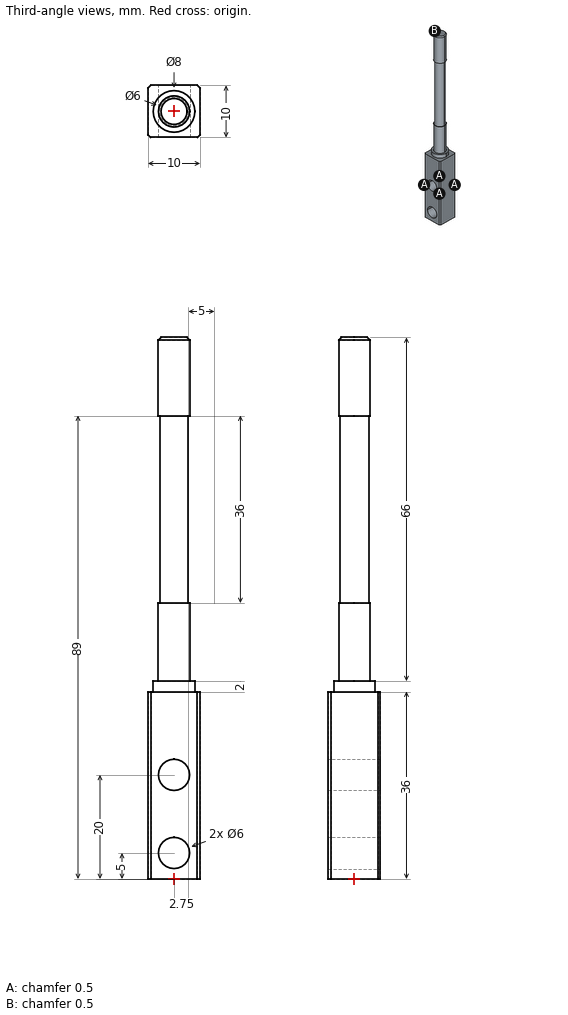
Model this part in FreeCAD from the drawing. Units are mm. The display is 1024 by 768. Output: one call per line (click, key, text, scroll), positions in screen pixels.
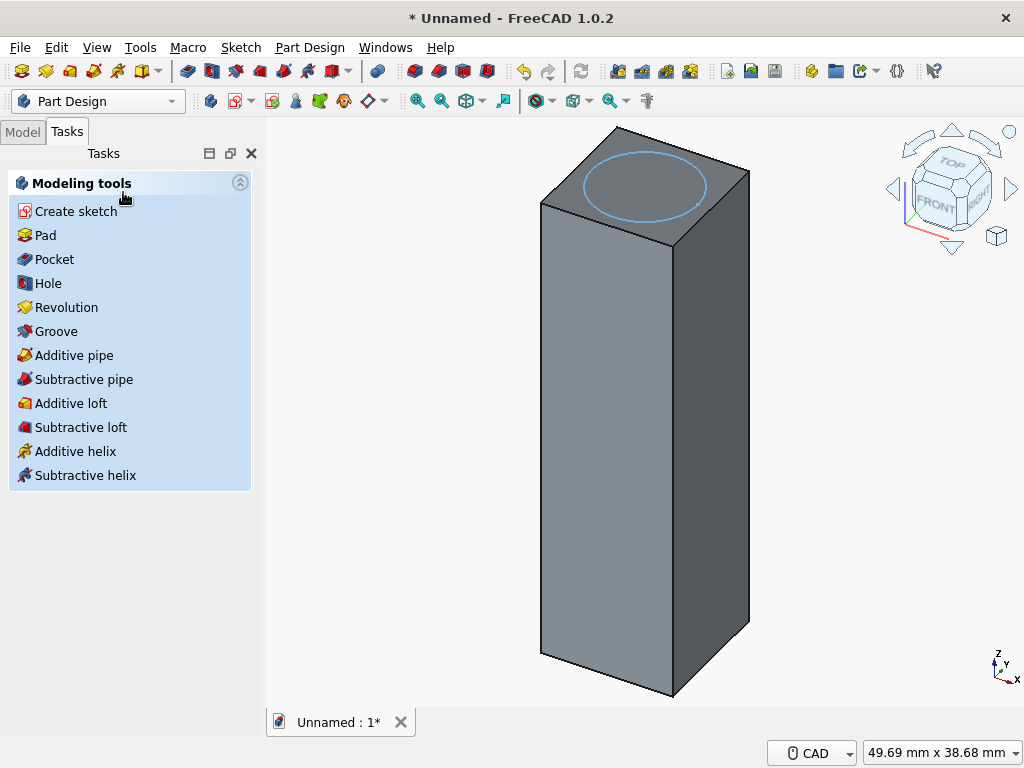
click(22, 72)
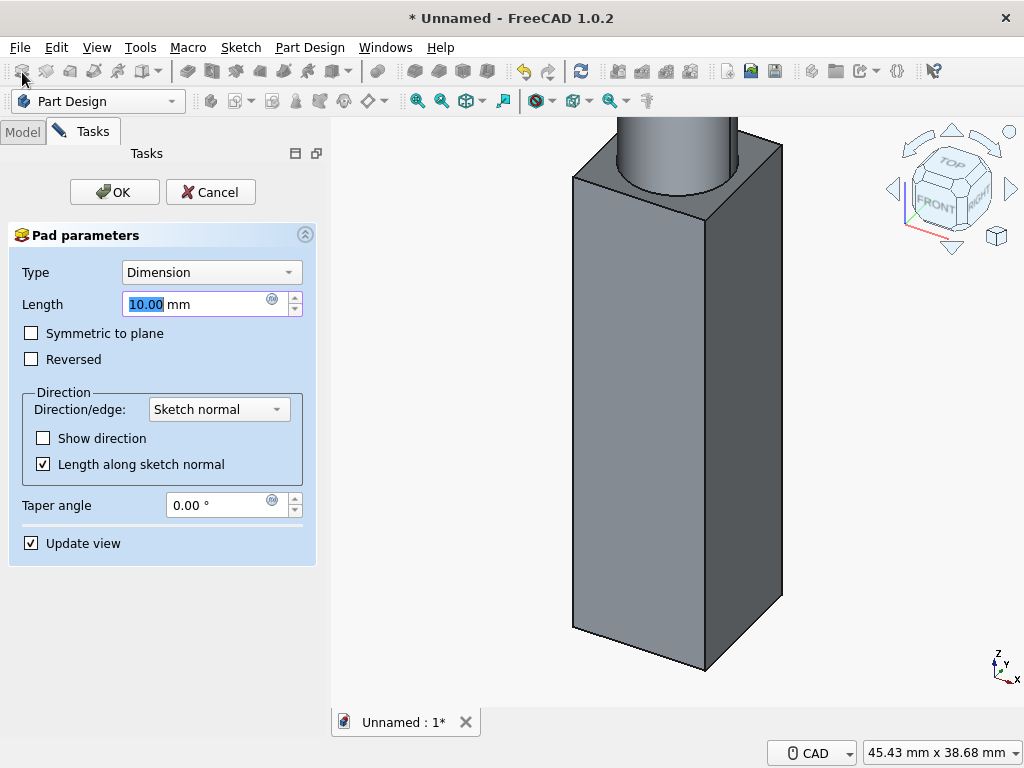
text(2)
key(Tab)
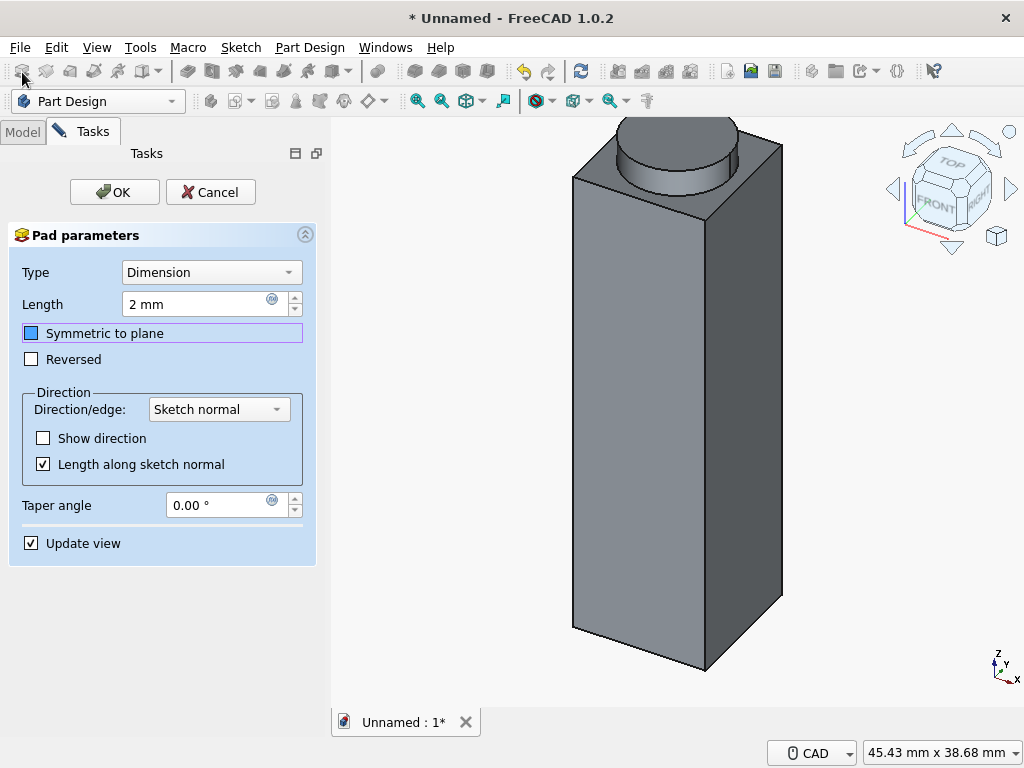
click(115, 192)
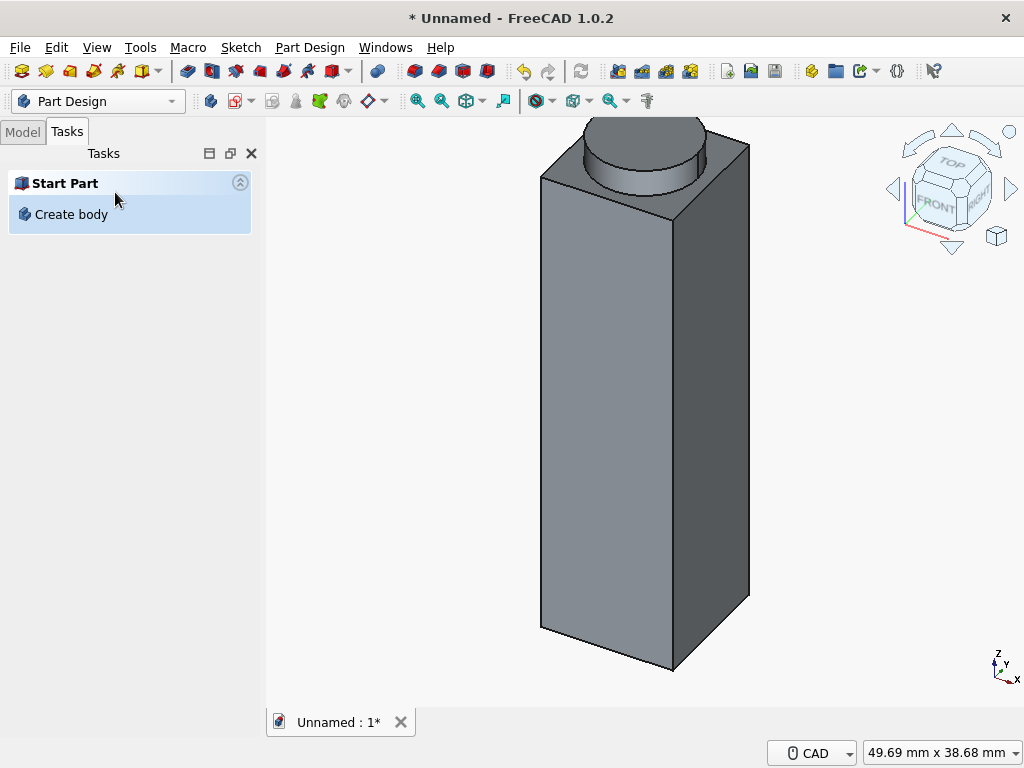
click(418, 102)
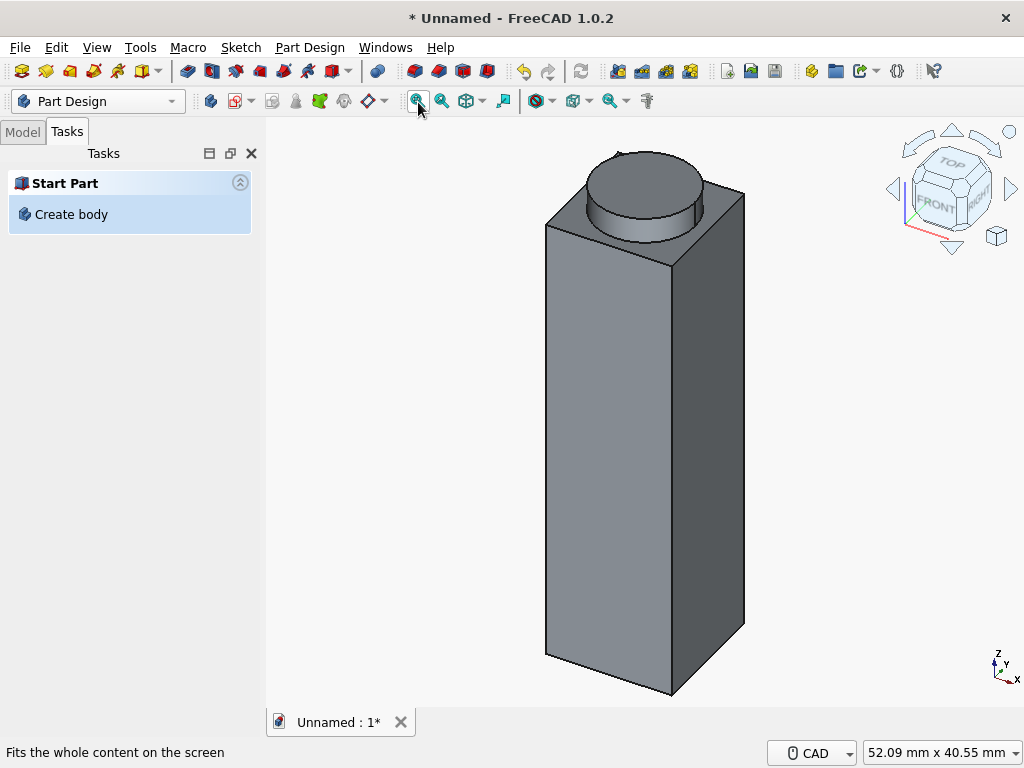
click(645, 185)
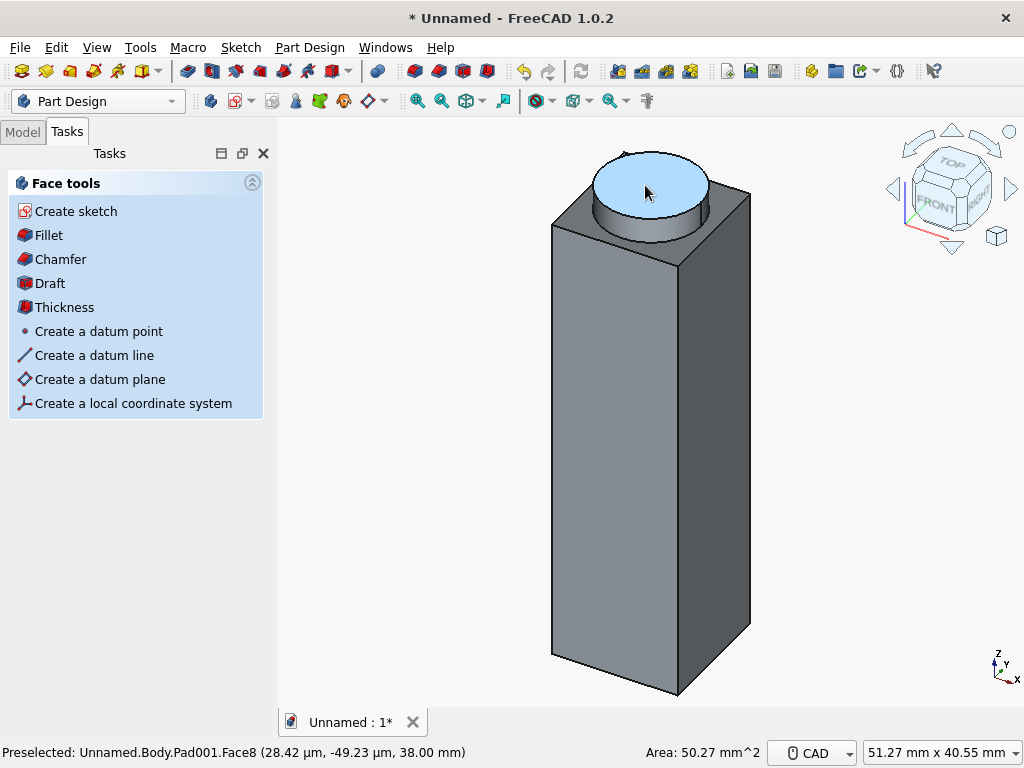
click(236, 102)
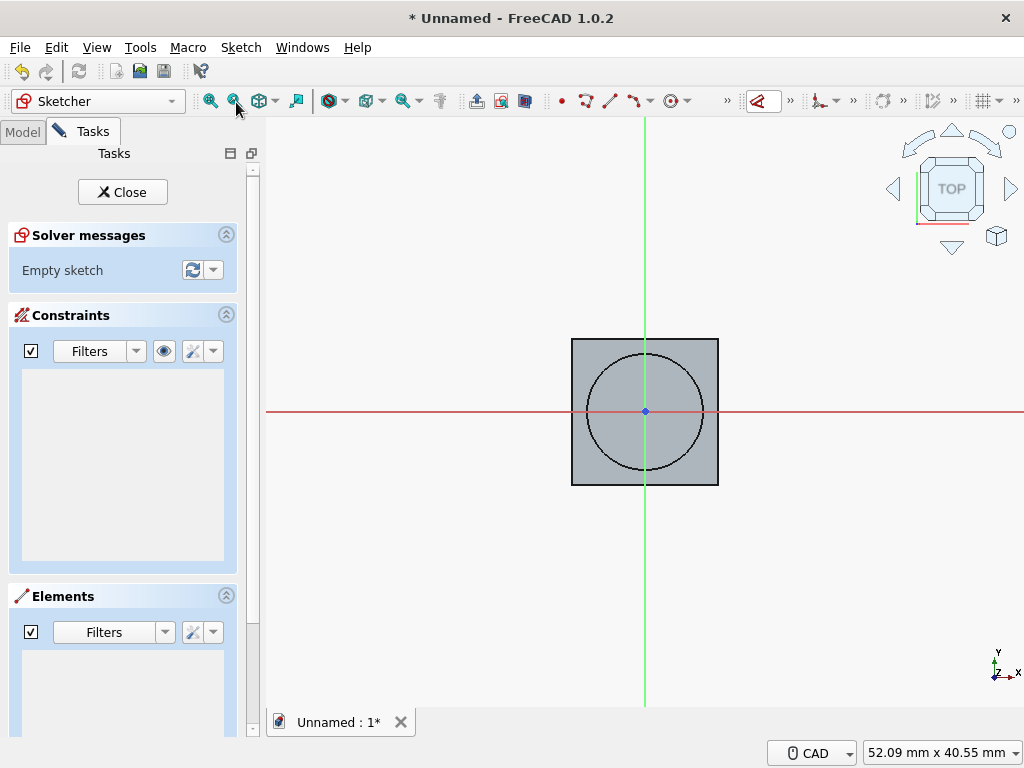
scroll(667, 412, up, 7)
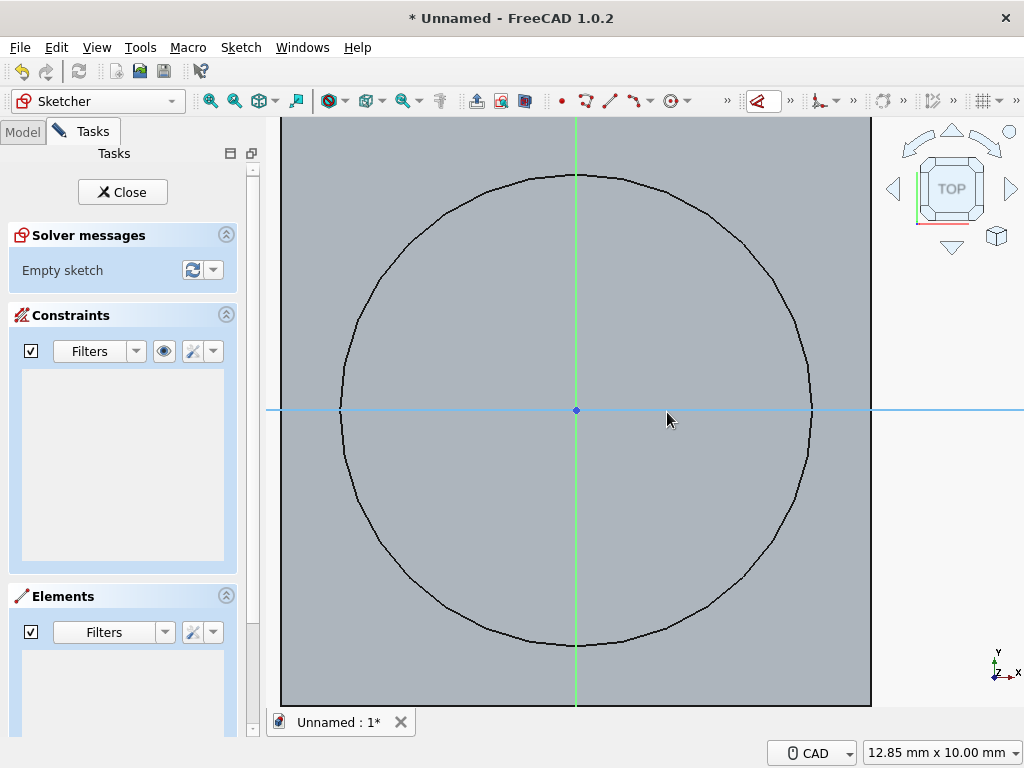
key(g)
key(c)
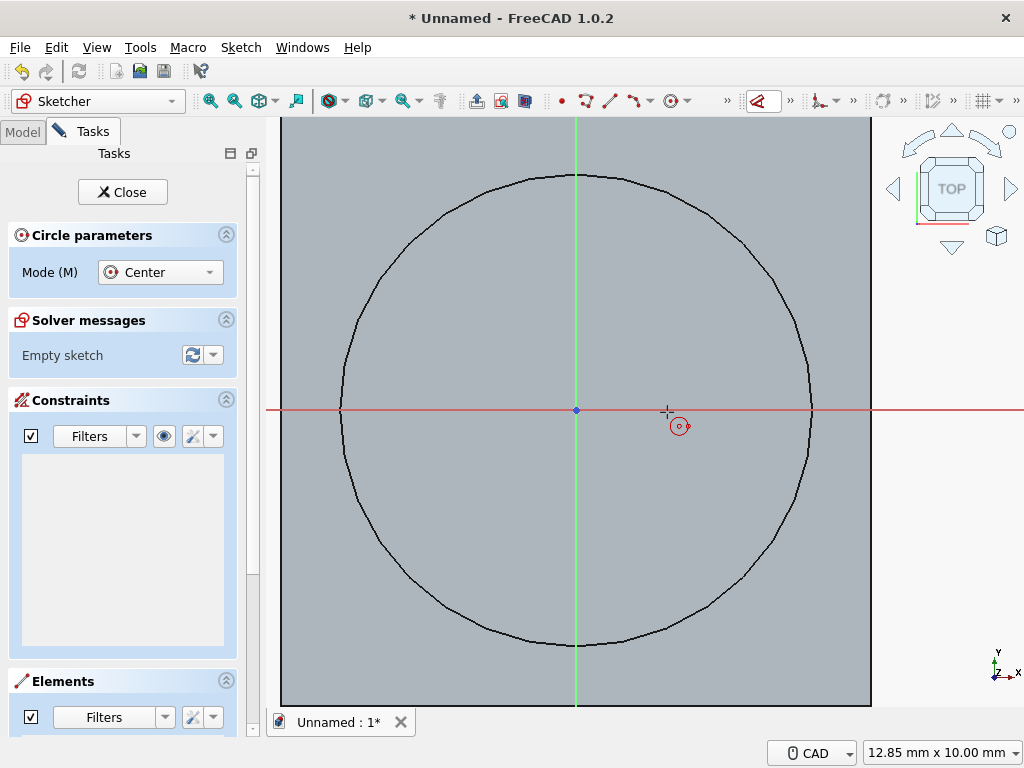
click(576, 410)
click(701, 285)
key(Escape)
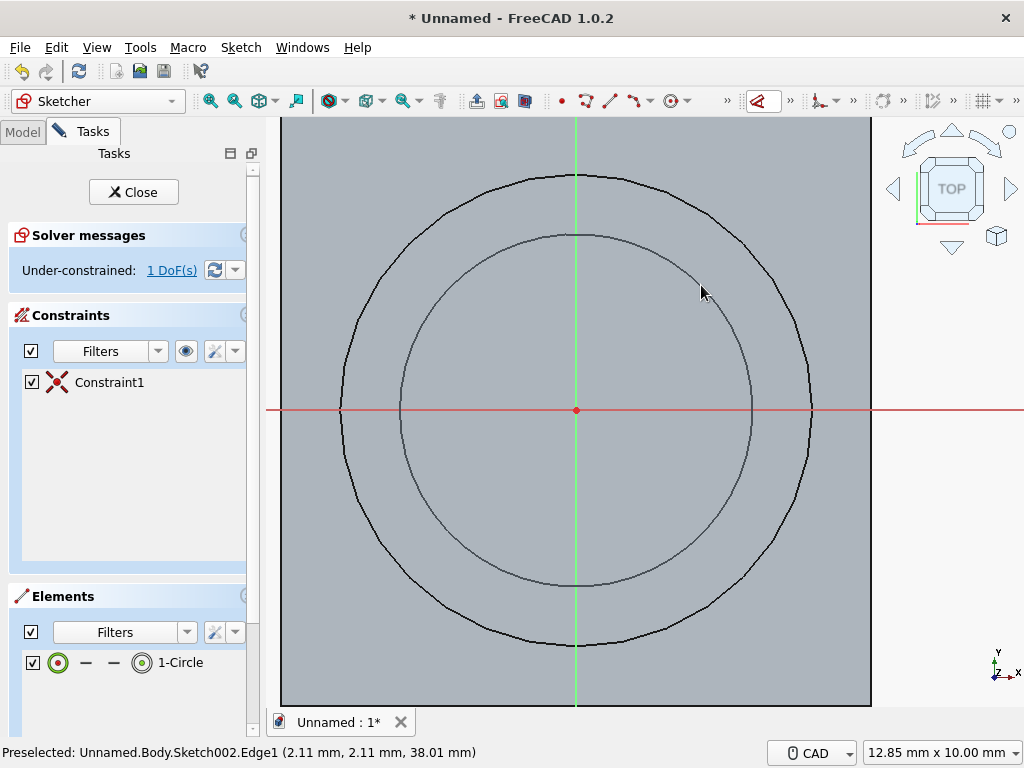
click(758, 102)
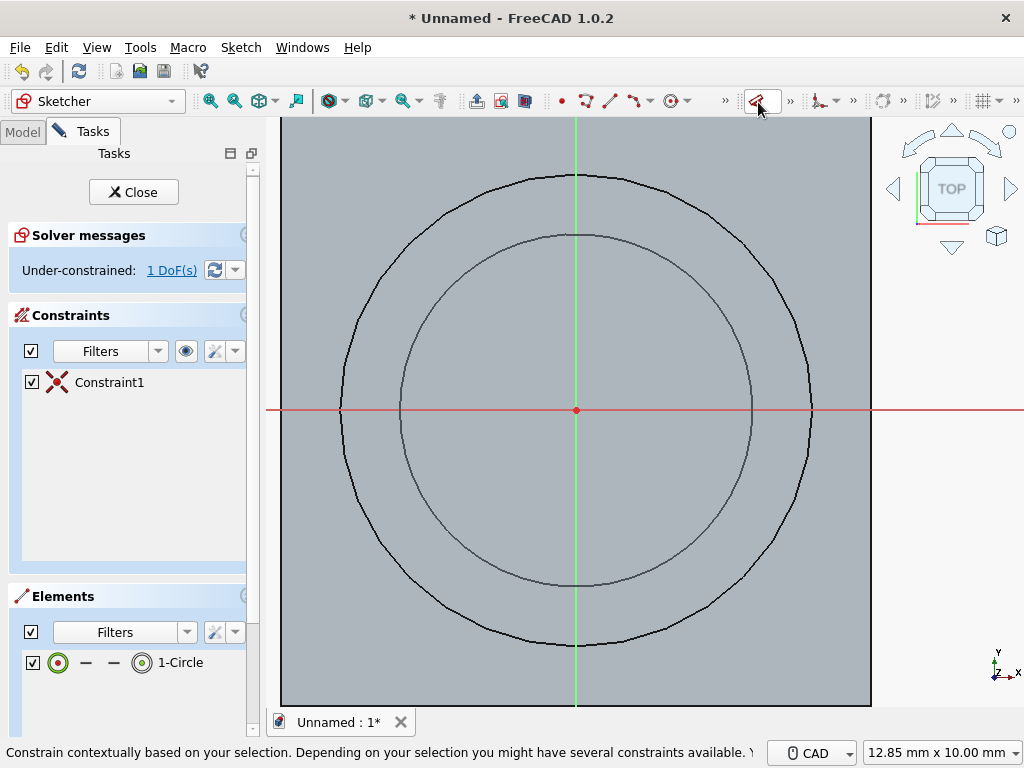
click(700, 285)
click(722, 262)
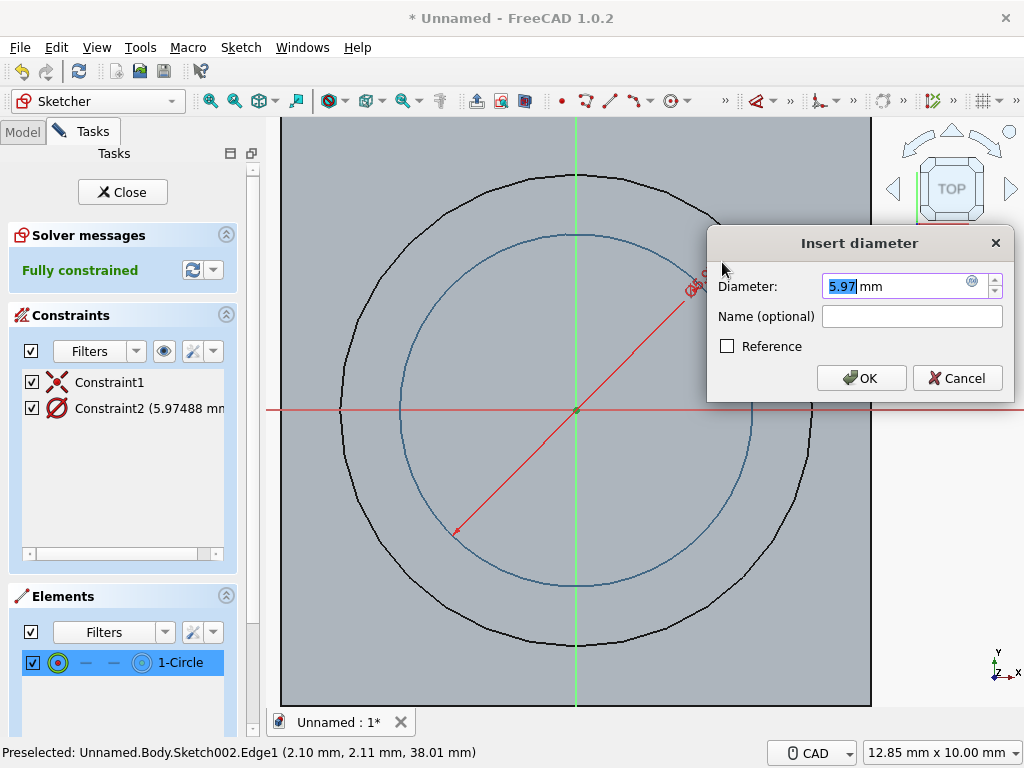
text(6)
key(Return)
key(Escape)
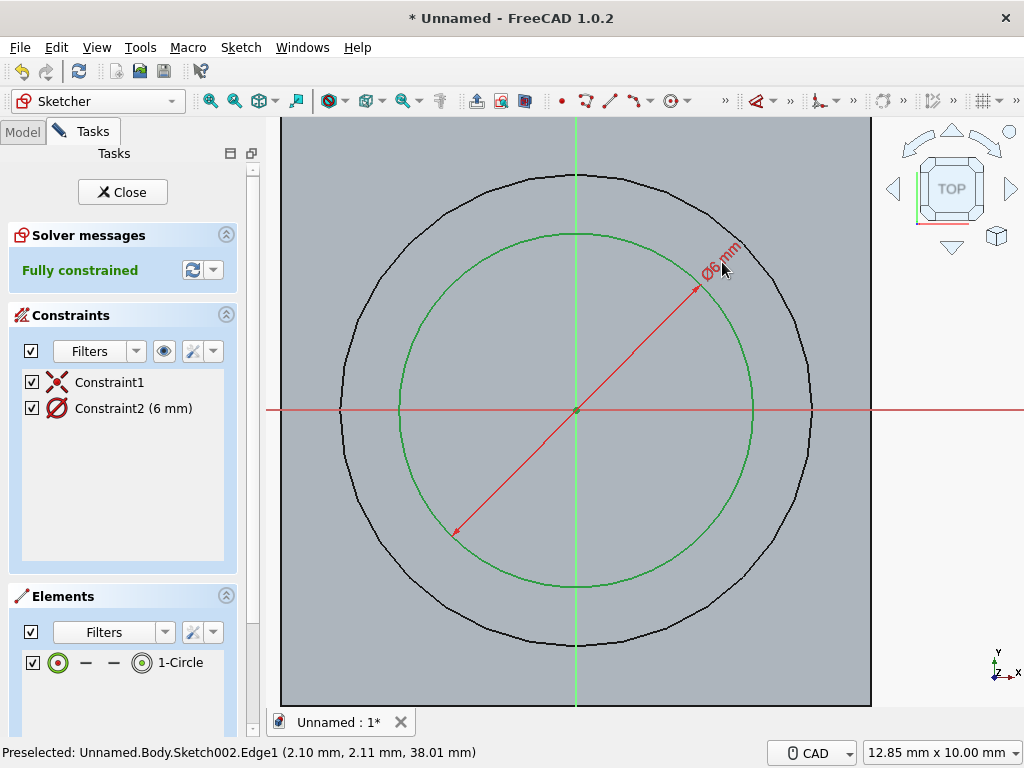
click(123, 192)